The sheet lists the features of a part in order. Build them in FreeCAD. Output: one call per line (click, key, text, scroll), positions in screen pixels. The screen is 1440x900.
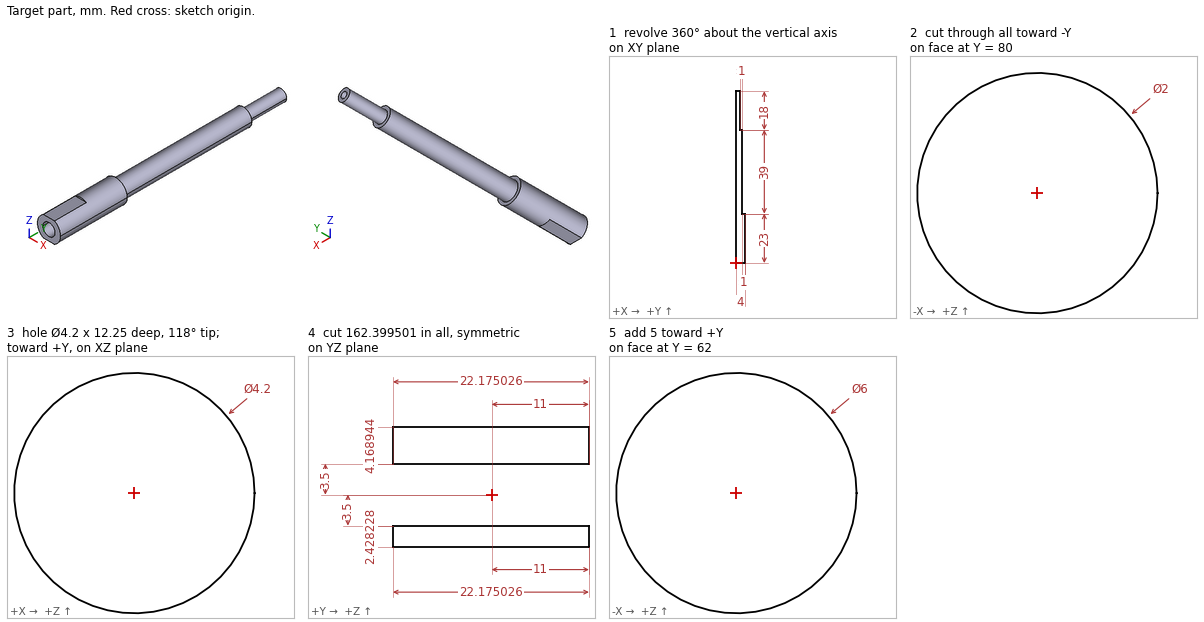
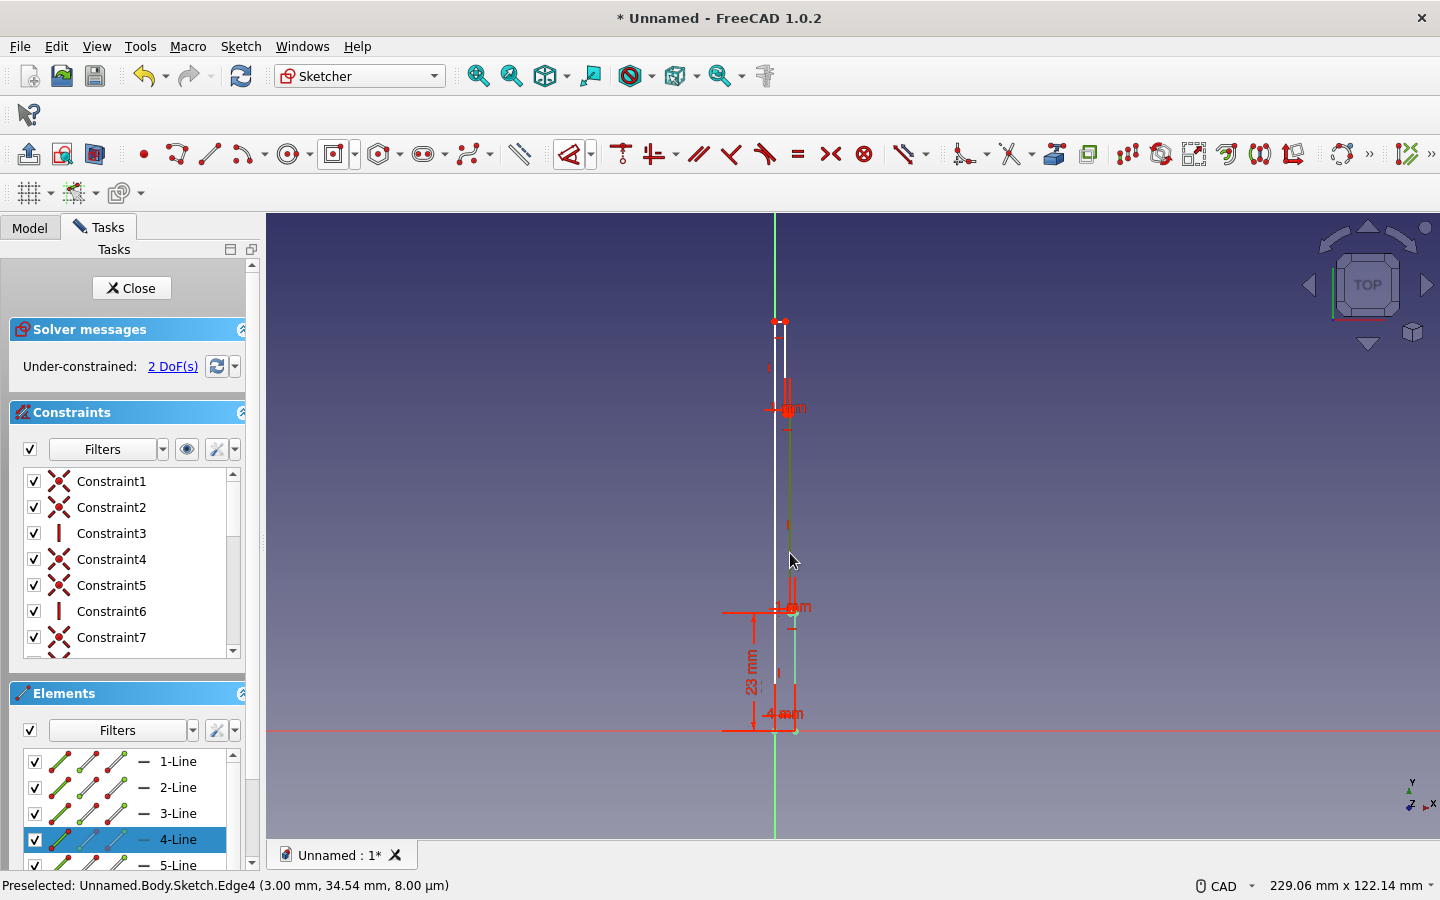
key(i)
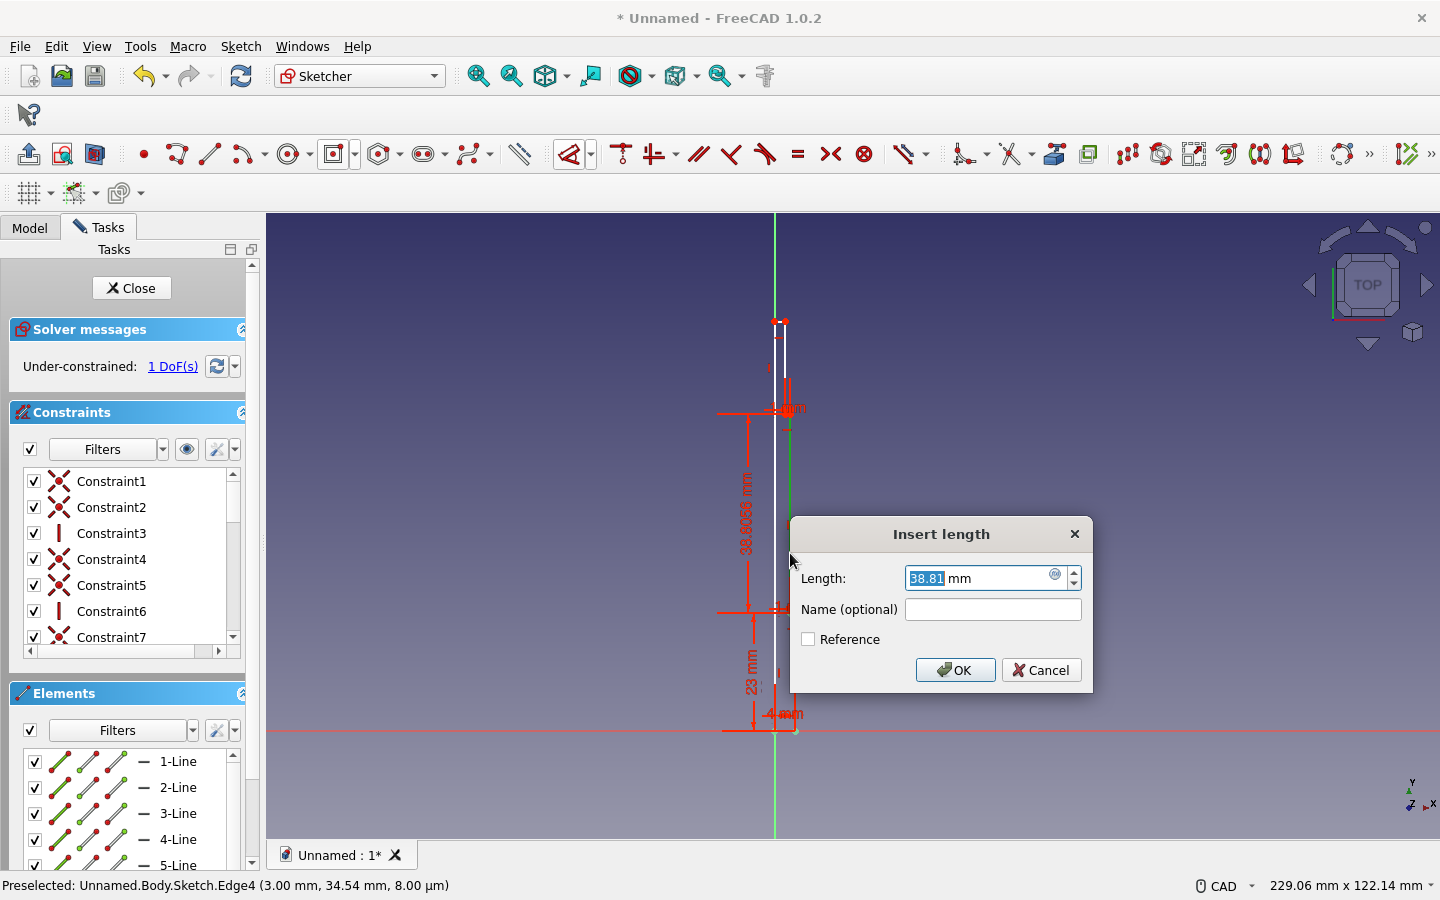
text(39)
key(Return)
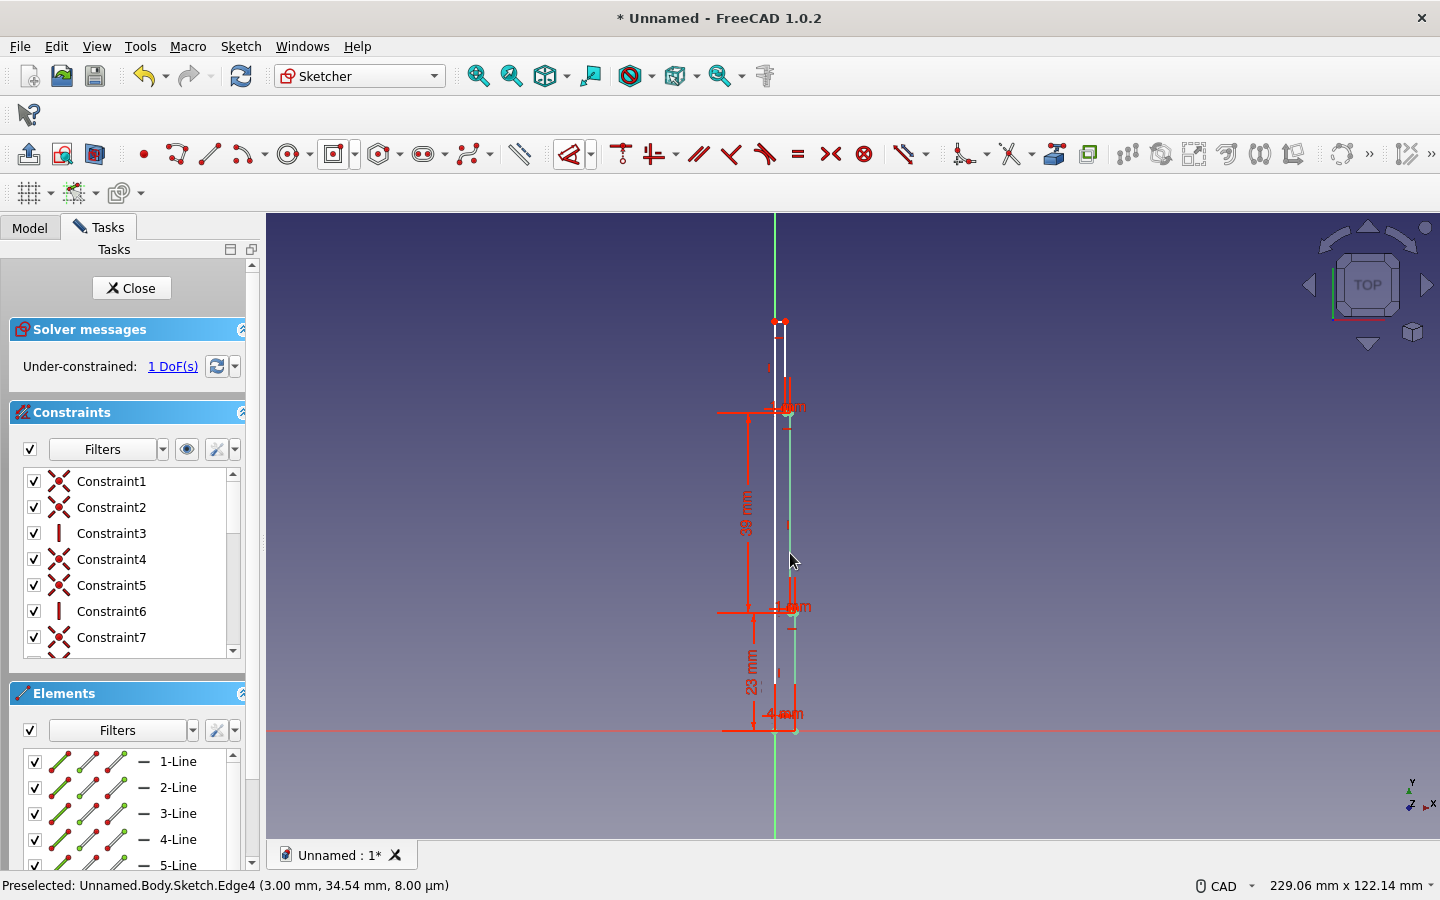
scroll(785, 386, up, 2)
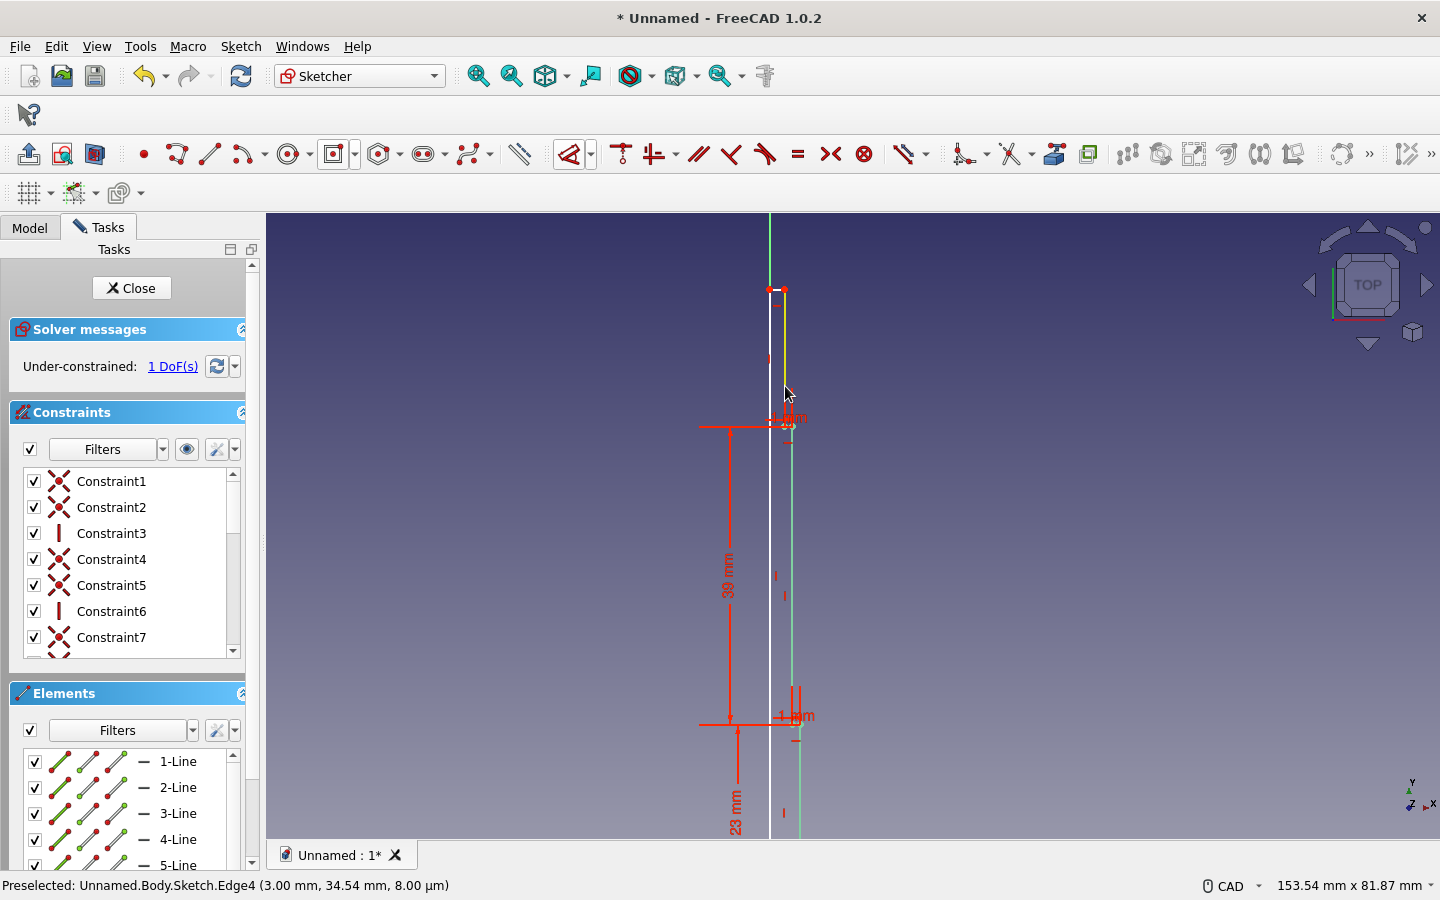
click(785, 386)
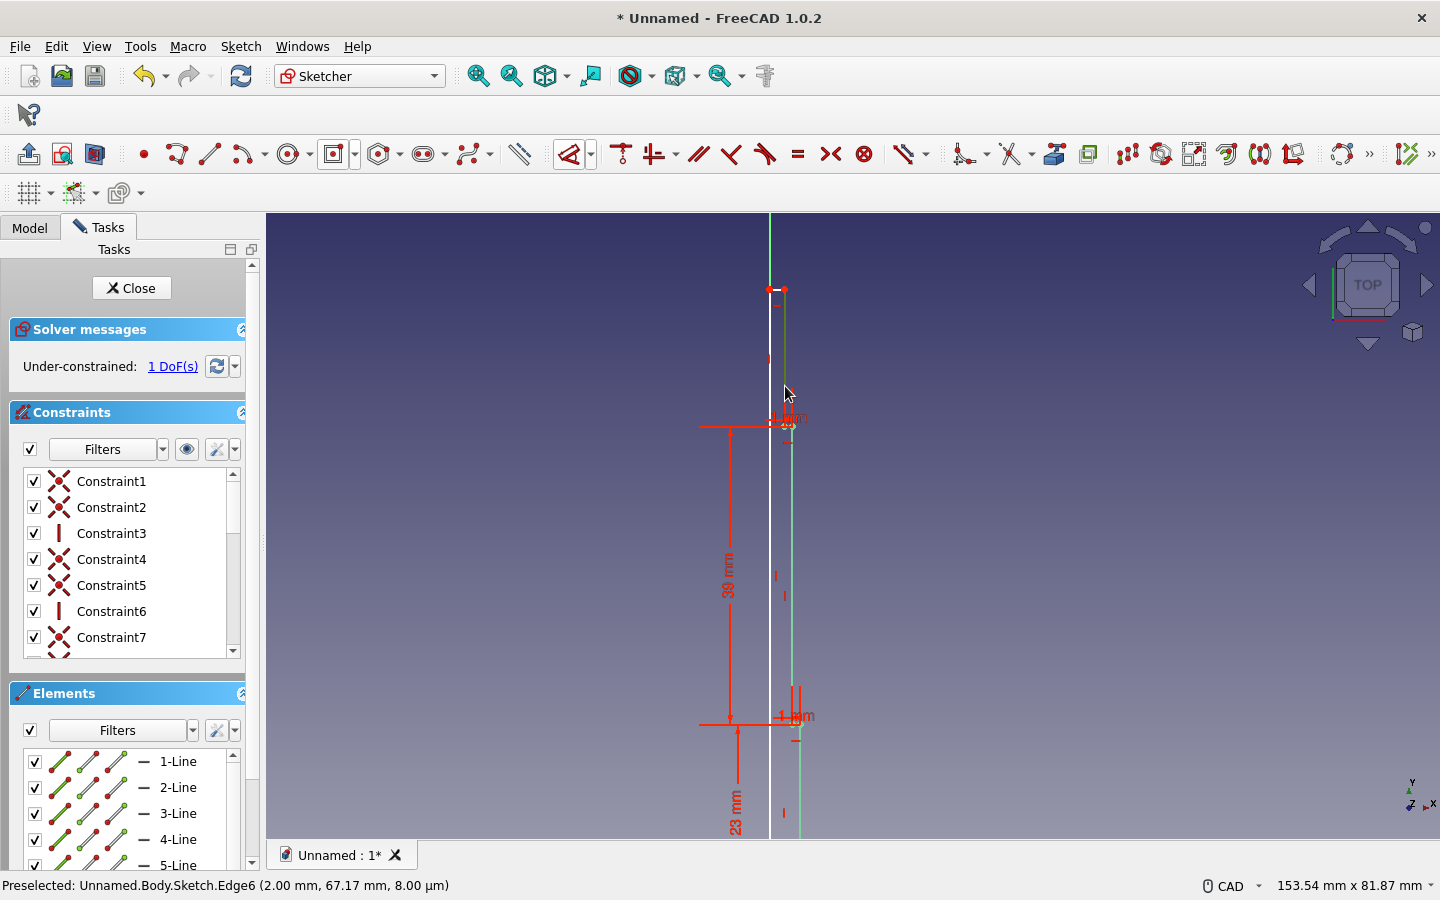
key(i)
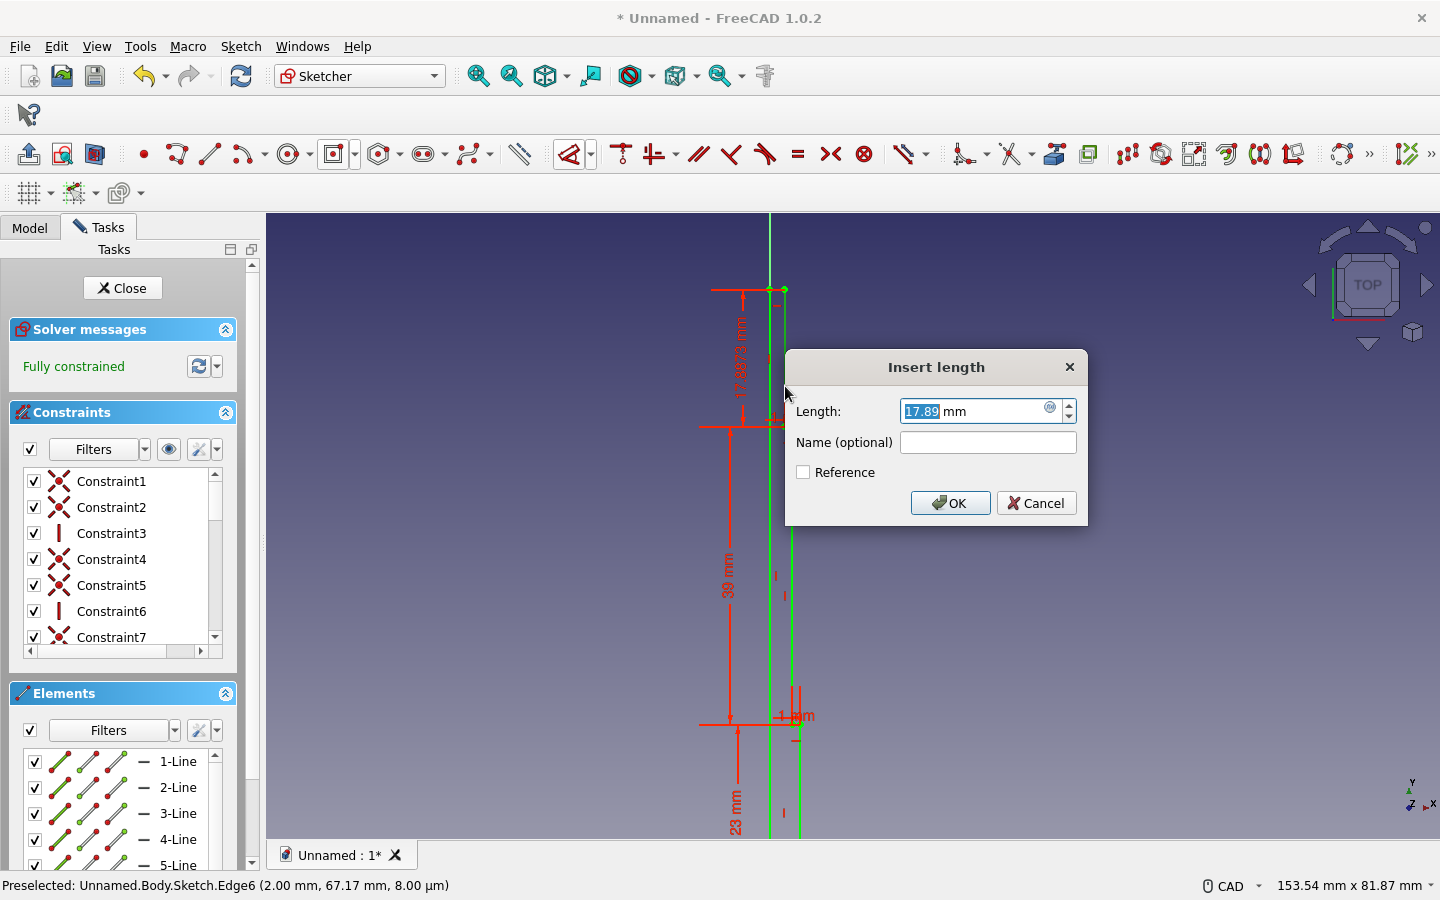
text(18)
key(Return)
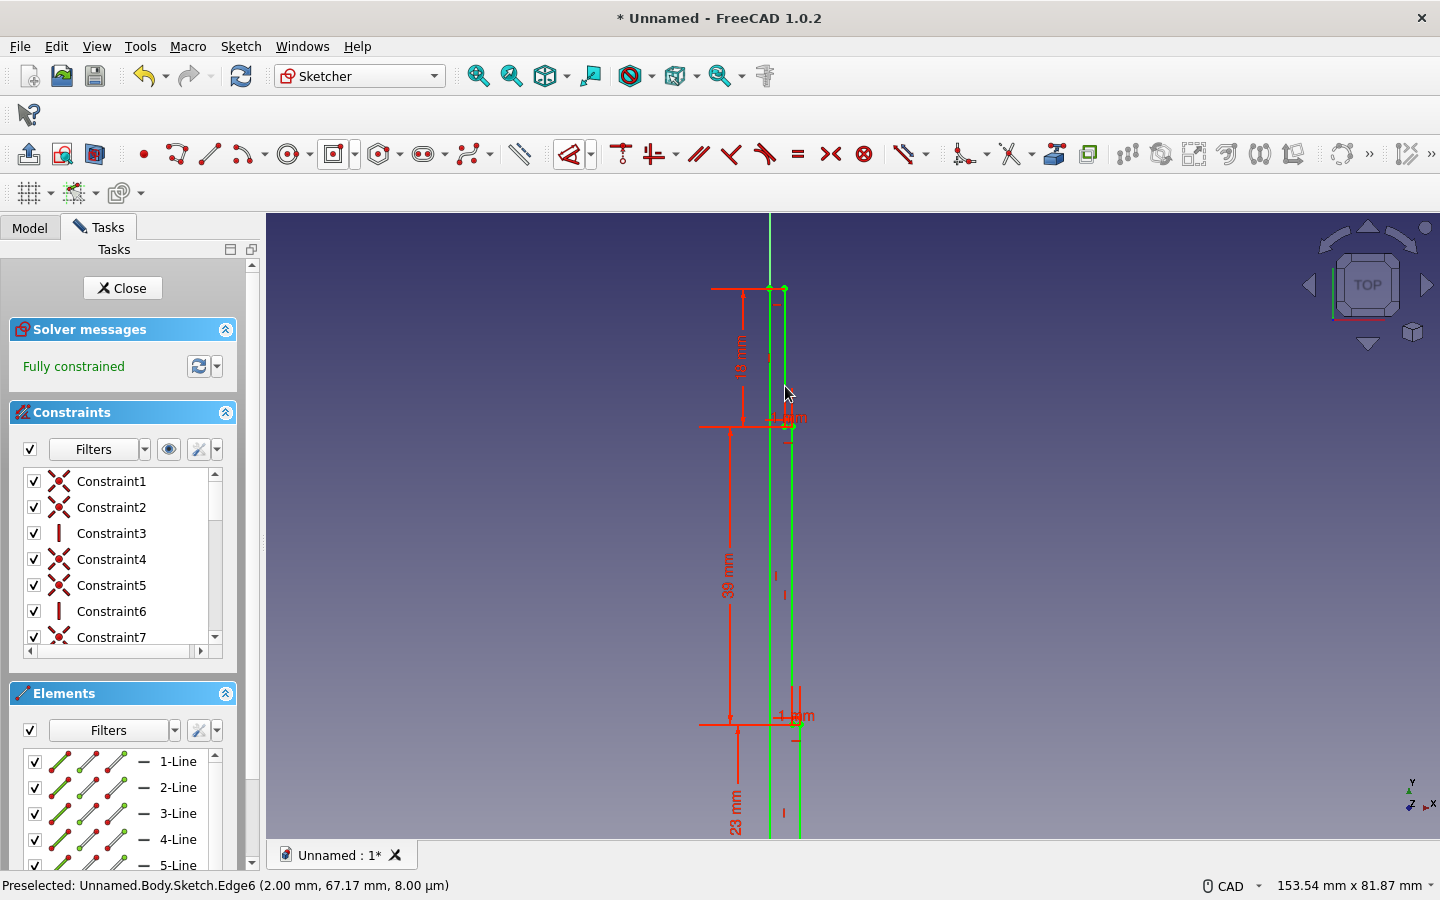
click(123, 288)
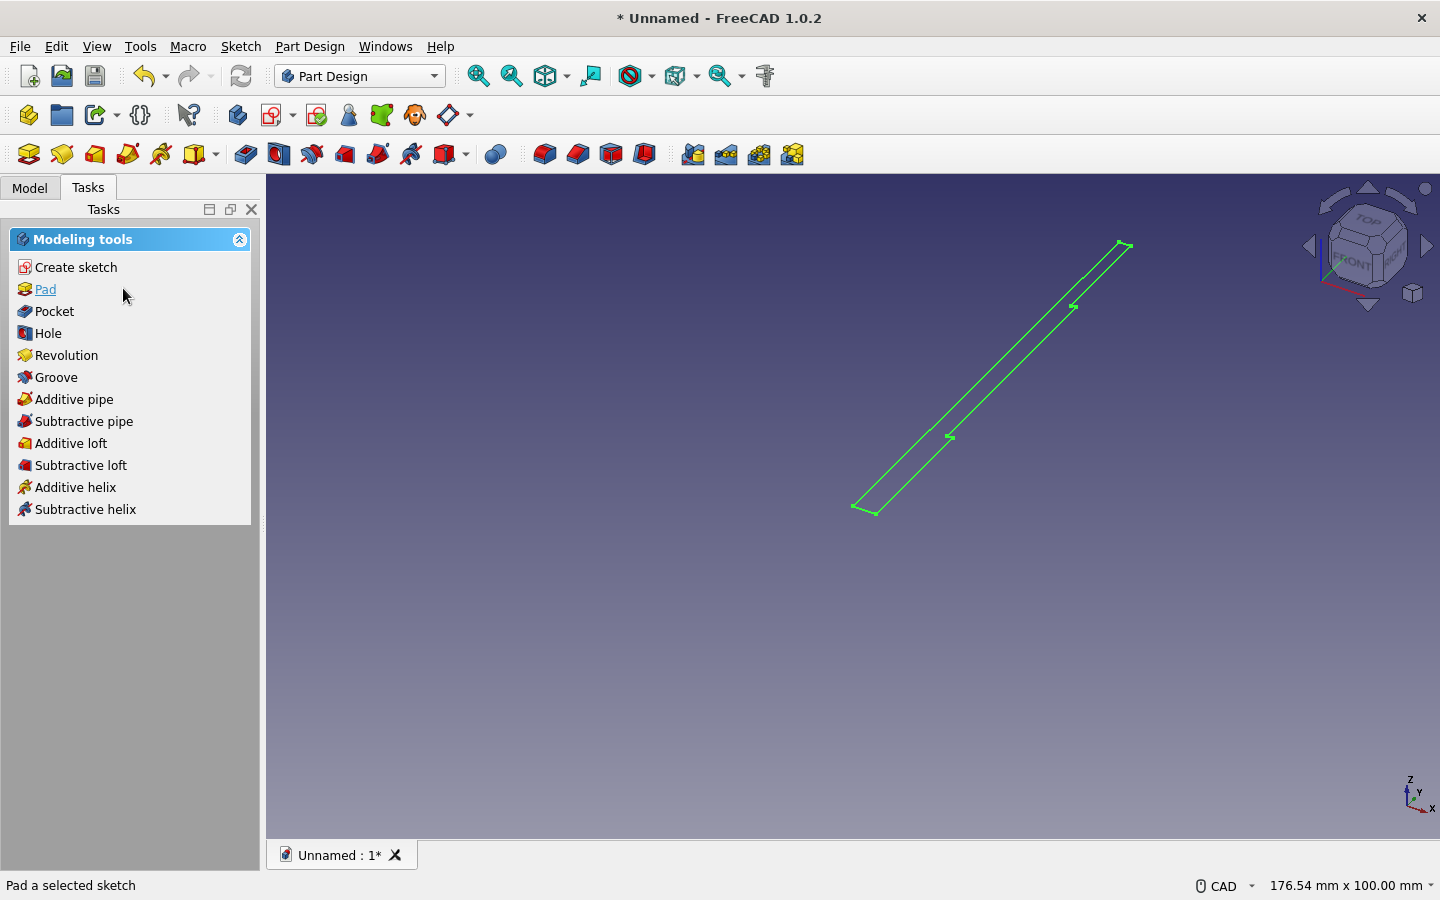
click(62, 154)